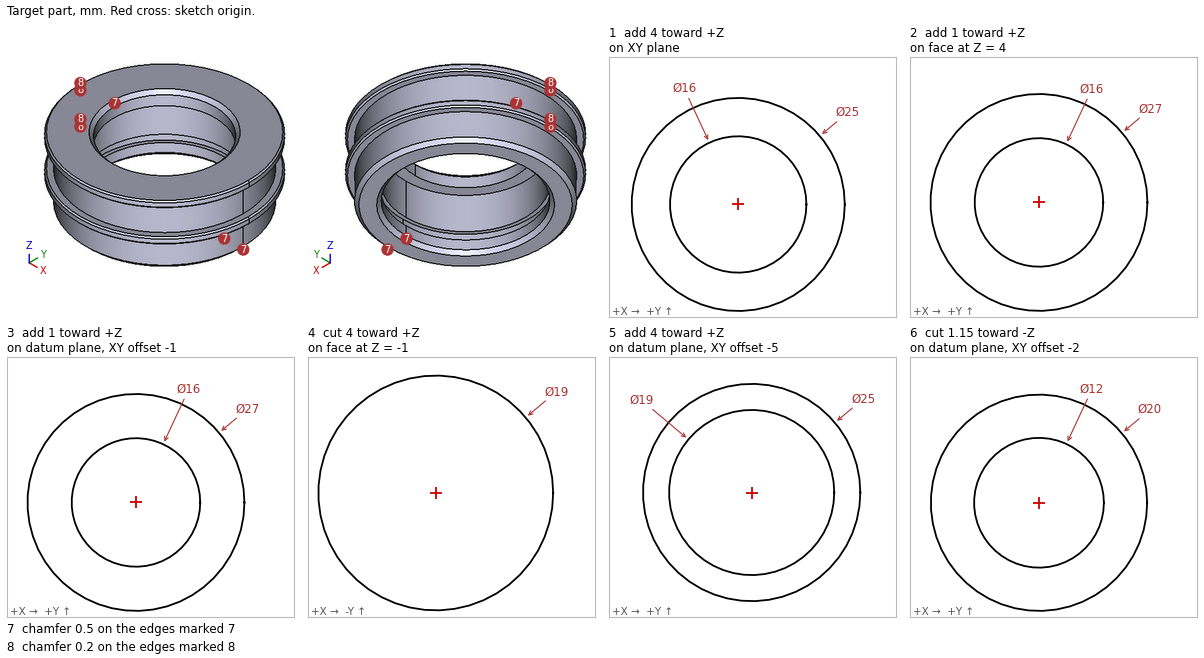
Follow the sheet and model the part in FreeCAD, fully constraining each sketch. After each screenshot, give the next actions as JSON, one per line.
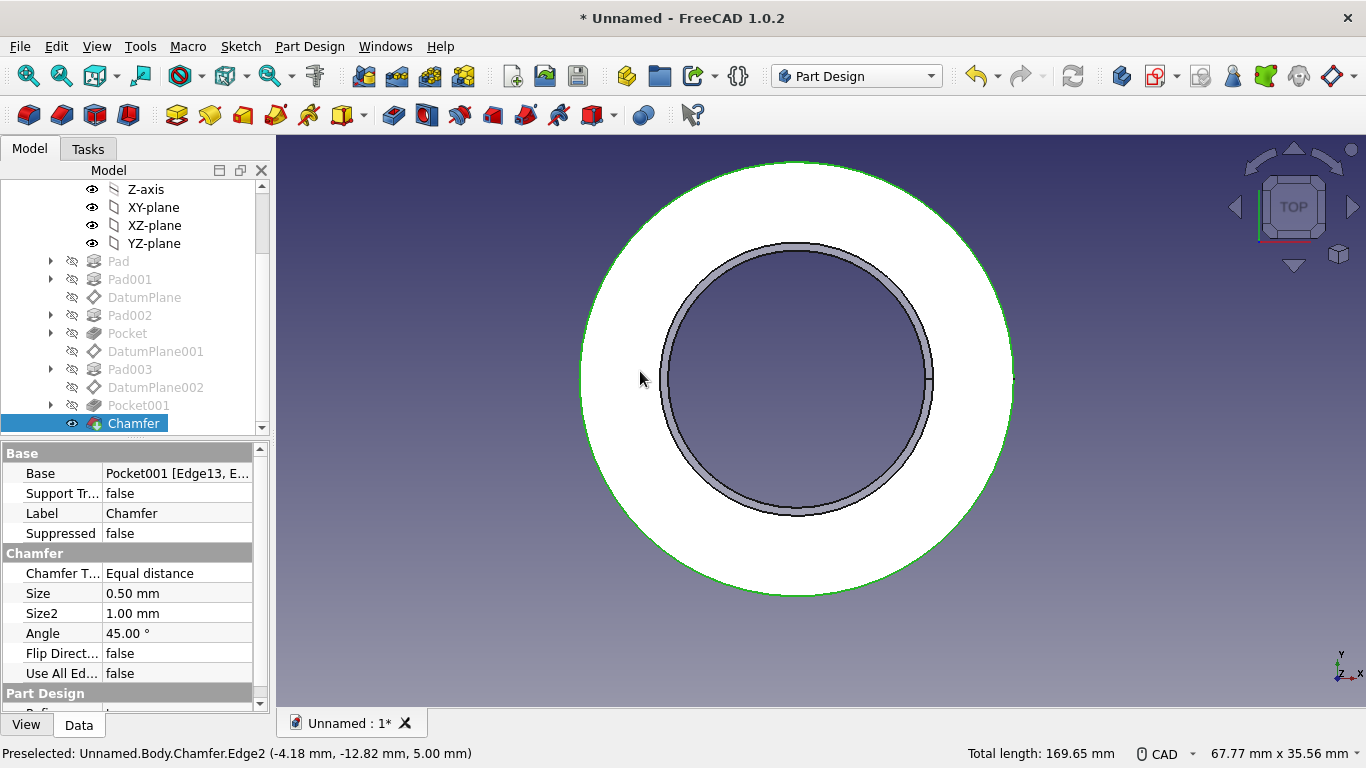
{"action": "key", "text": "0"}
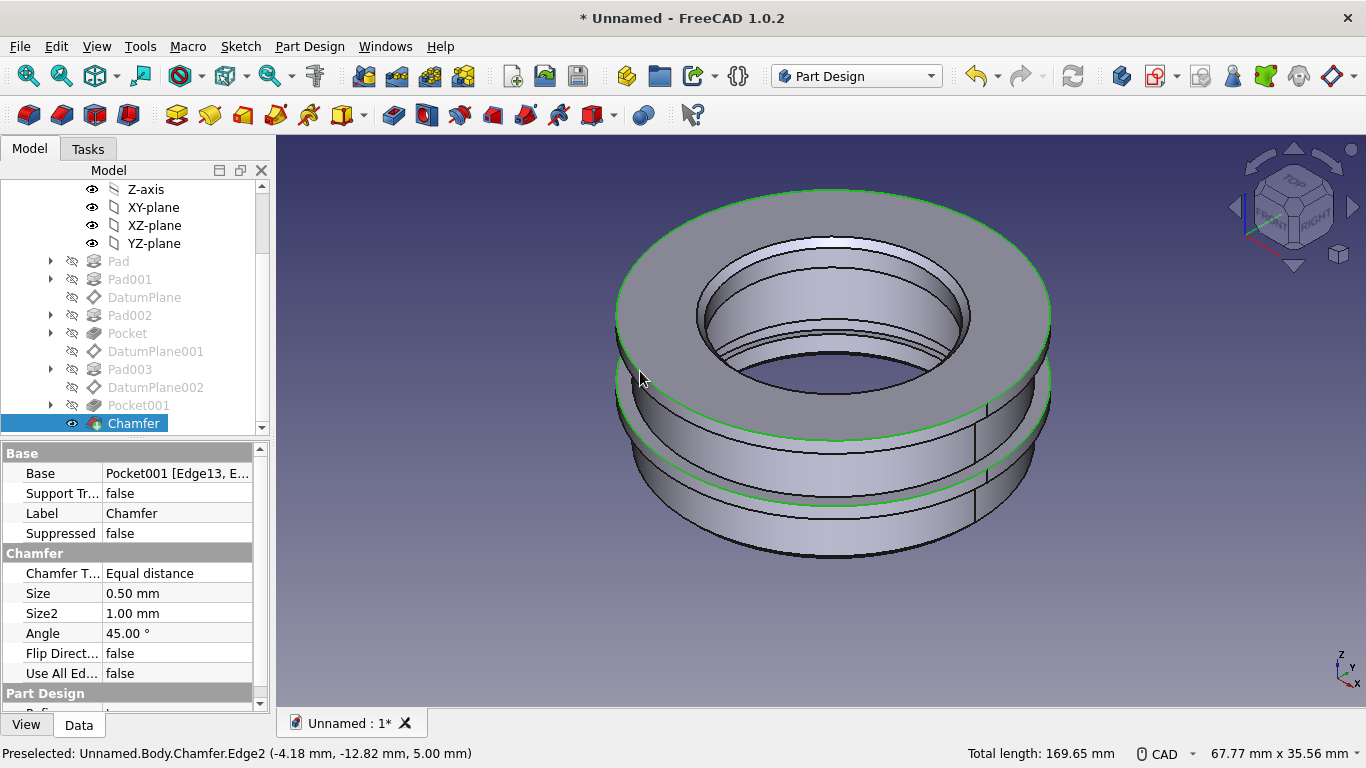
{"action": "key", "text": "1"}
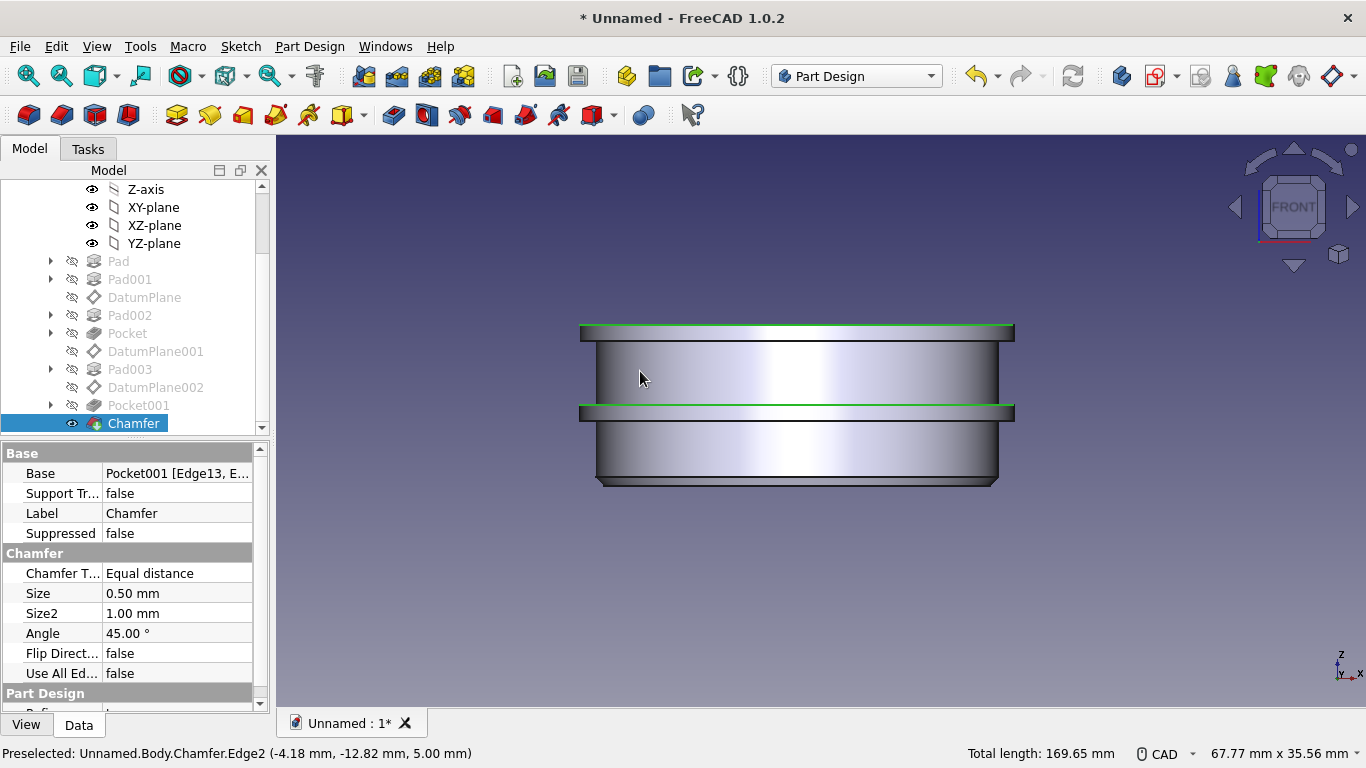
{"action": "left_click", "coordinate": [29, 76]}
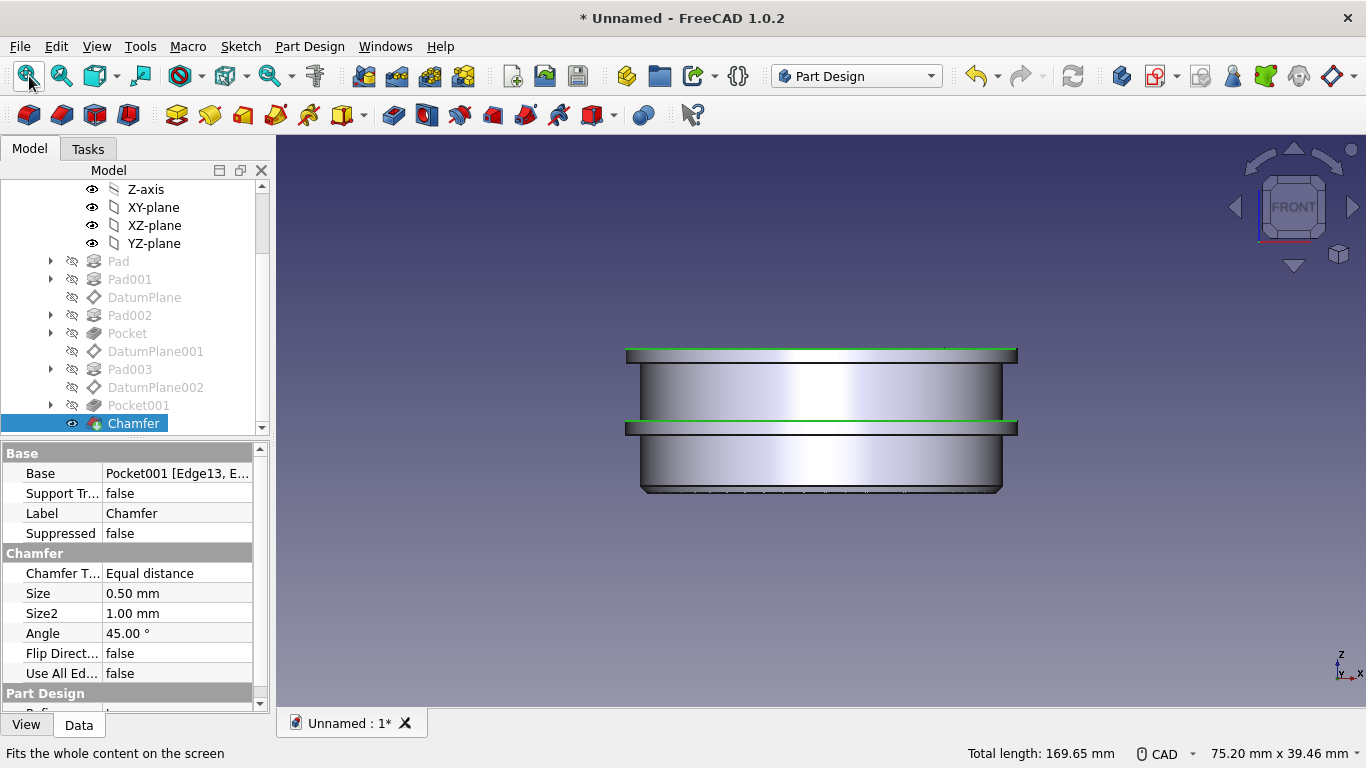
{"action": "left_click", "coordinate": [663, 362], "text": "ctrl"}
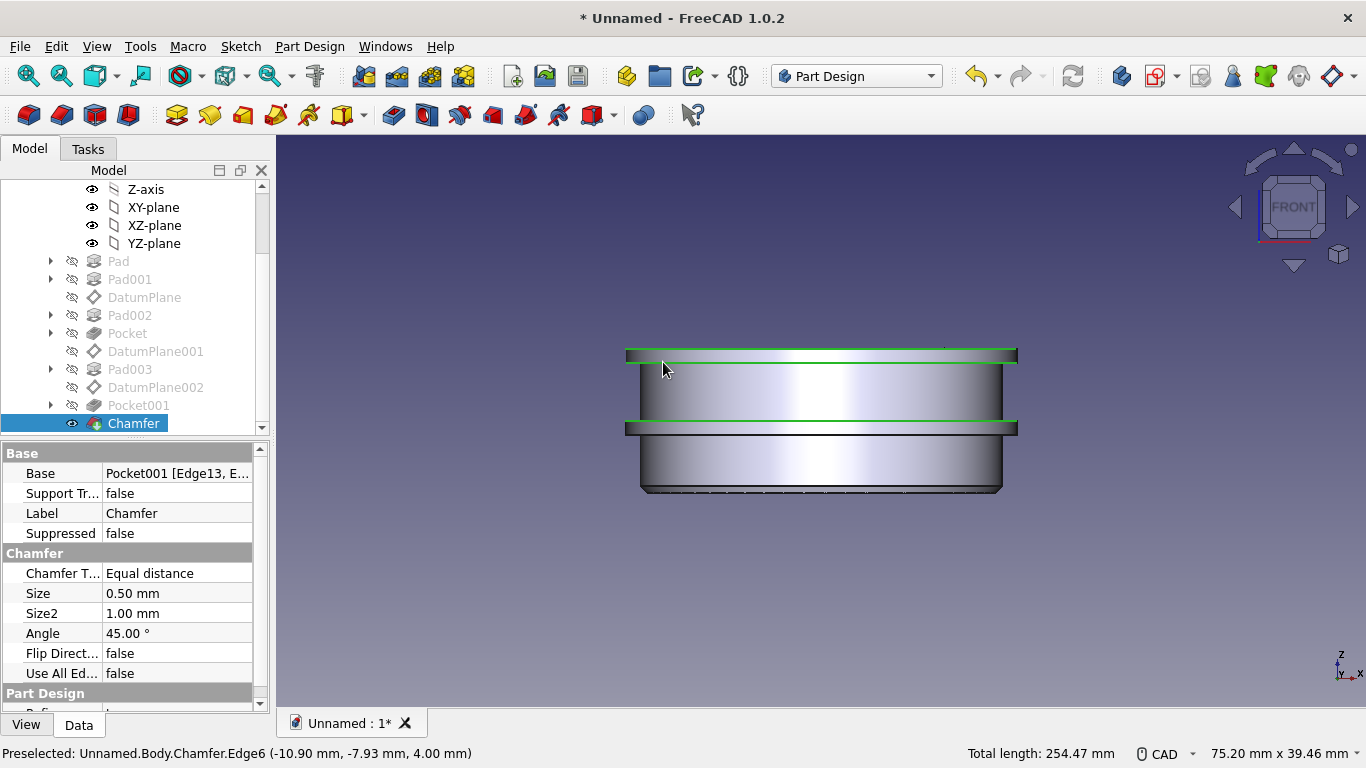
{"action": "left_click", "coordinate": [663, 434], "text": "ctrl"}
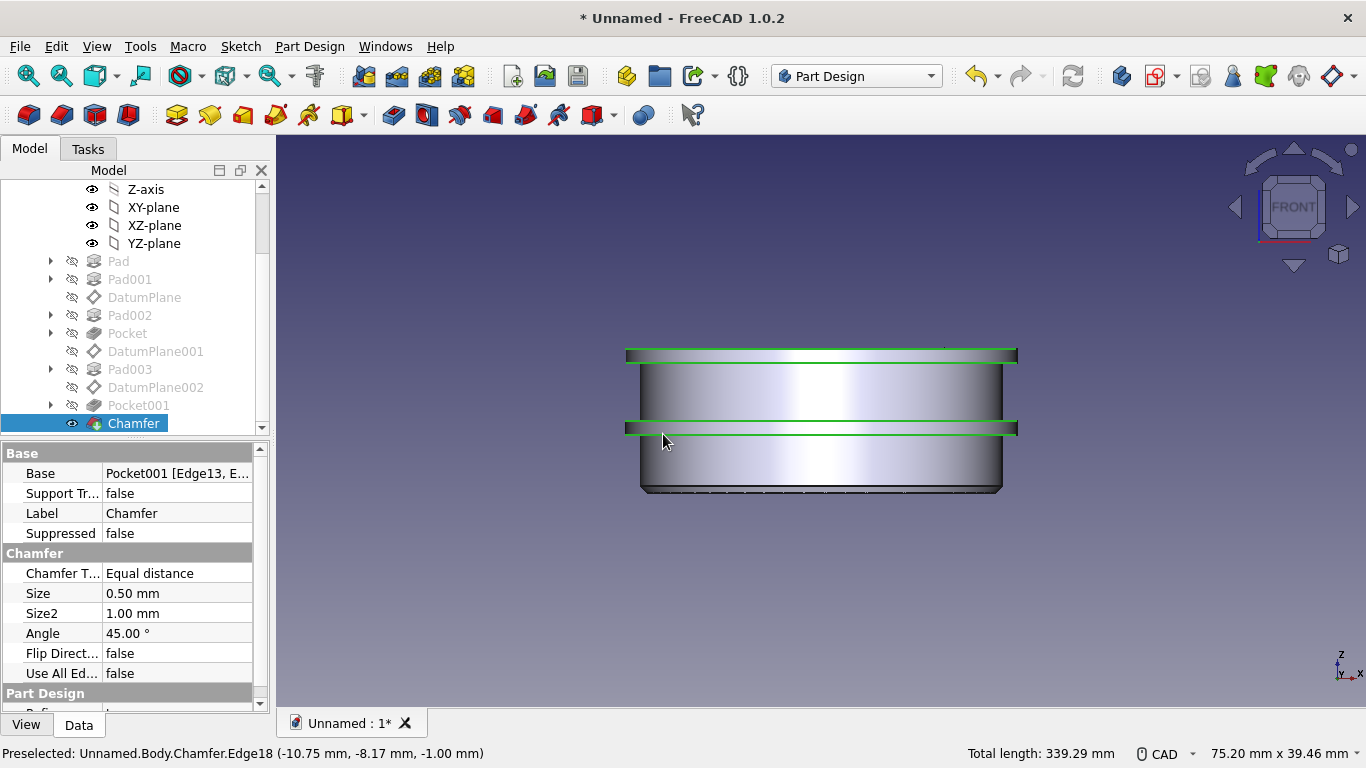
{"action": "left_click", "coordinate": [62, 116]}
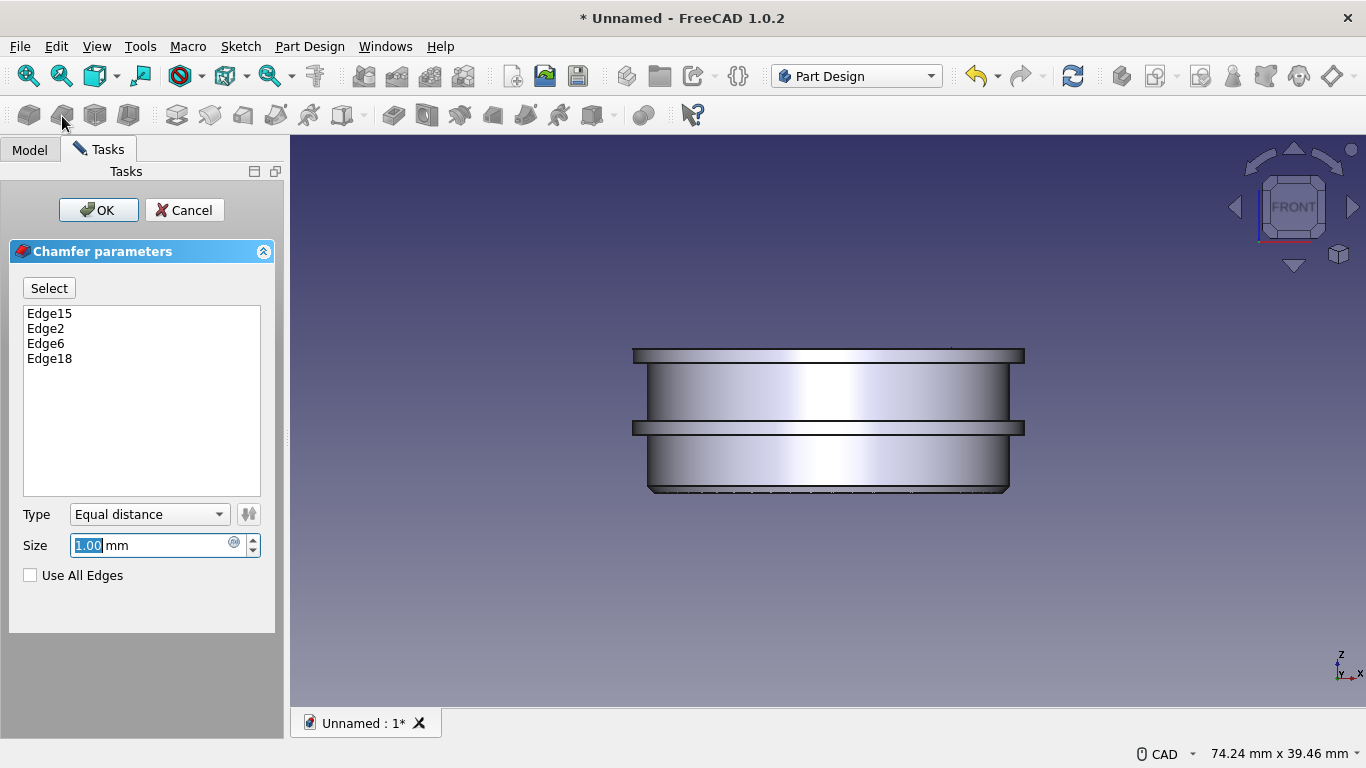
{"action": "type", "text": "0.2"}
{"action": "key", "text": "Tab"}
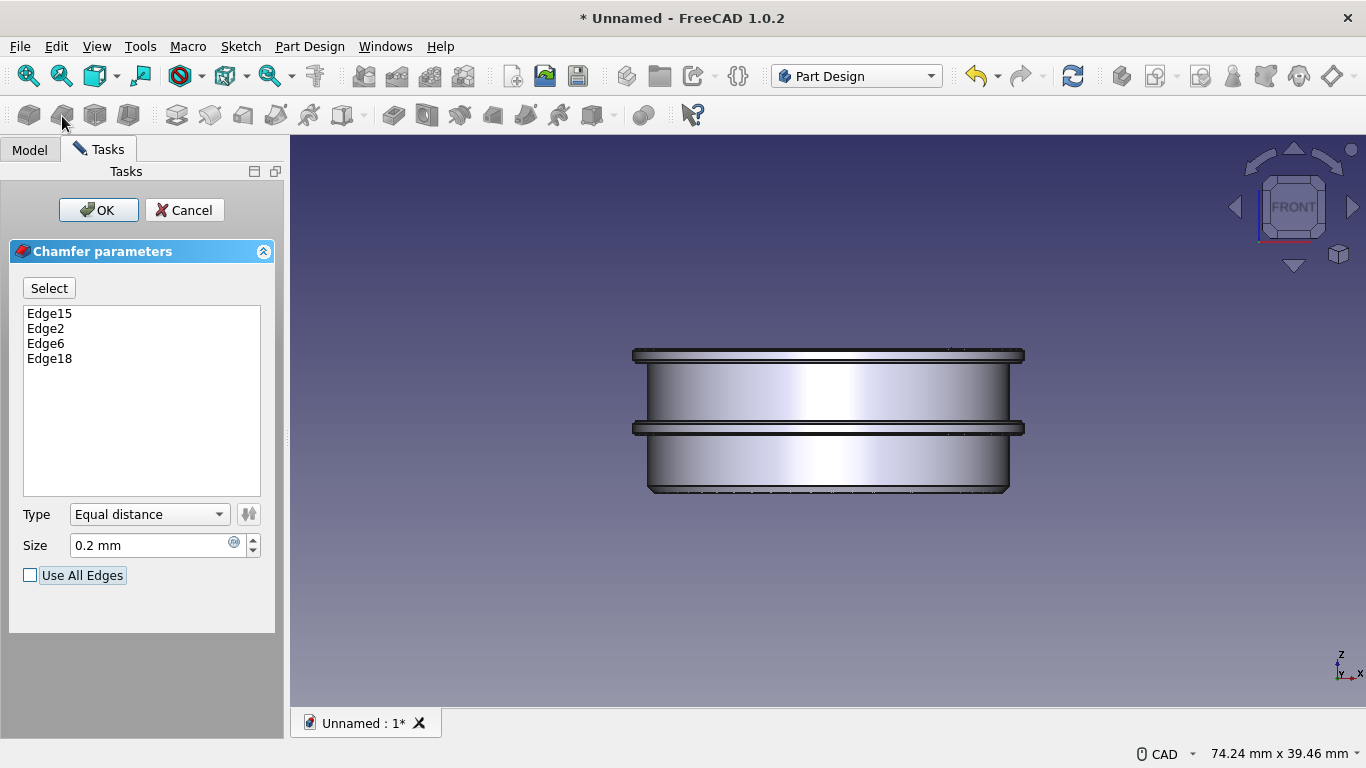
{"action": "left_click", "coordinate": [99, 210]}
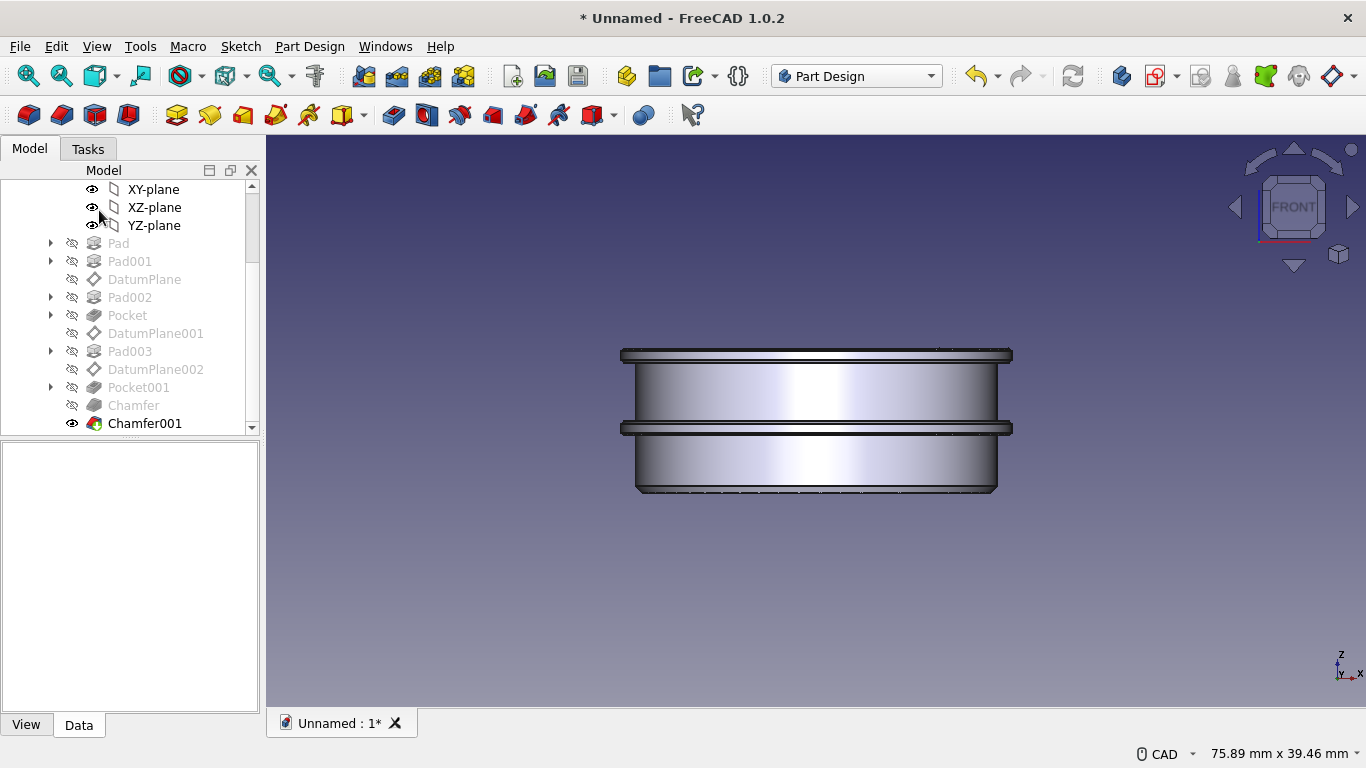
{"action": "key", "text": "0"}